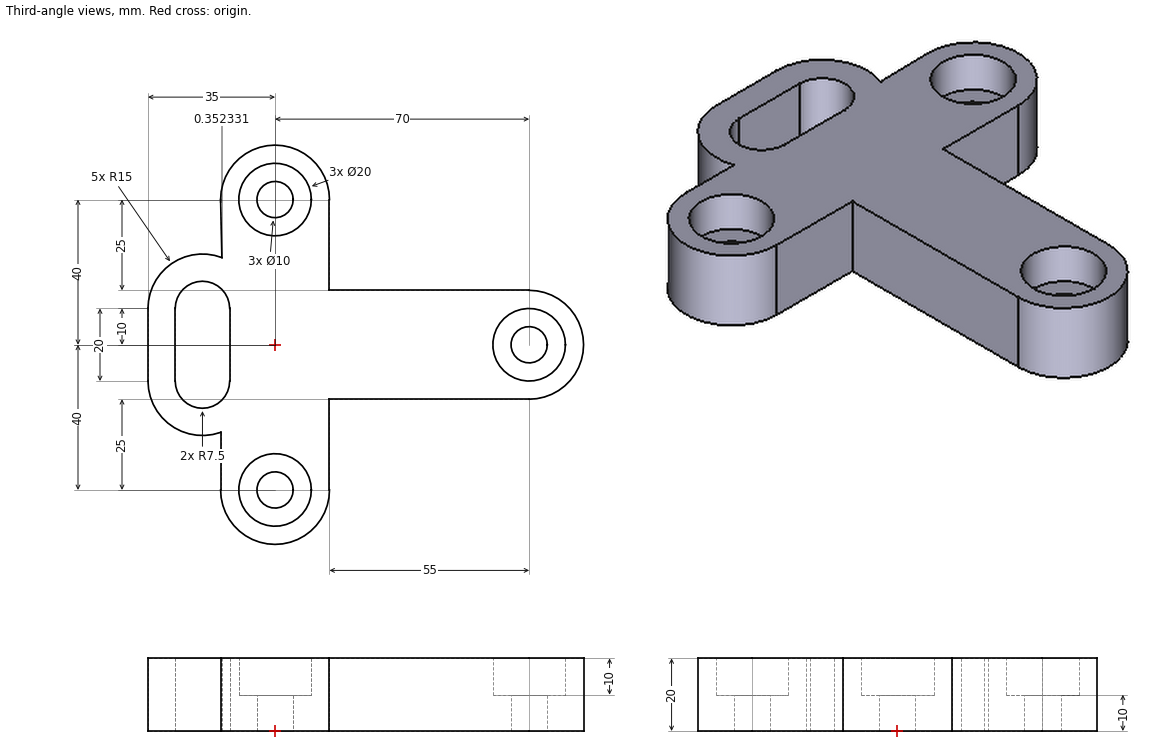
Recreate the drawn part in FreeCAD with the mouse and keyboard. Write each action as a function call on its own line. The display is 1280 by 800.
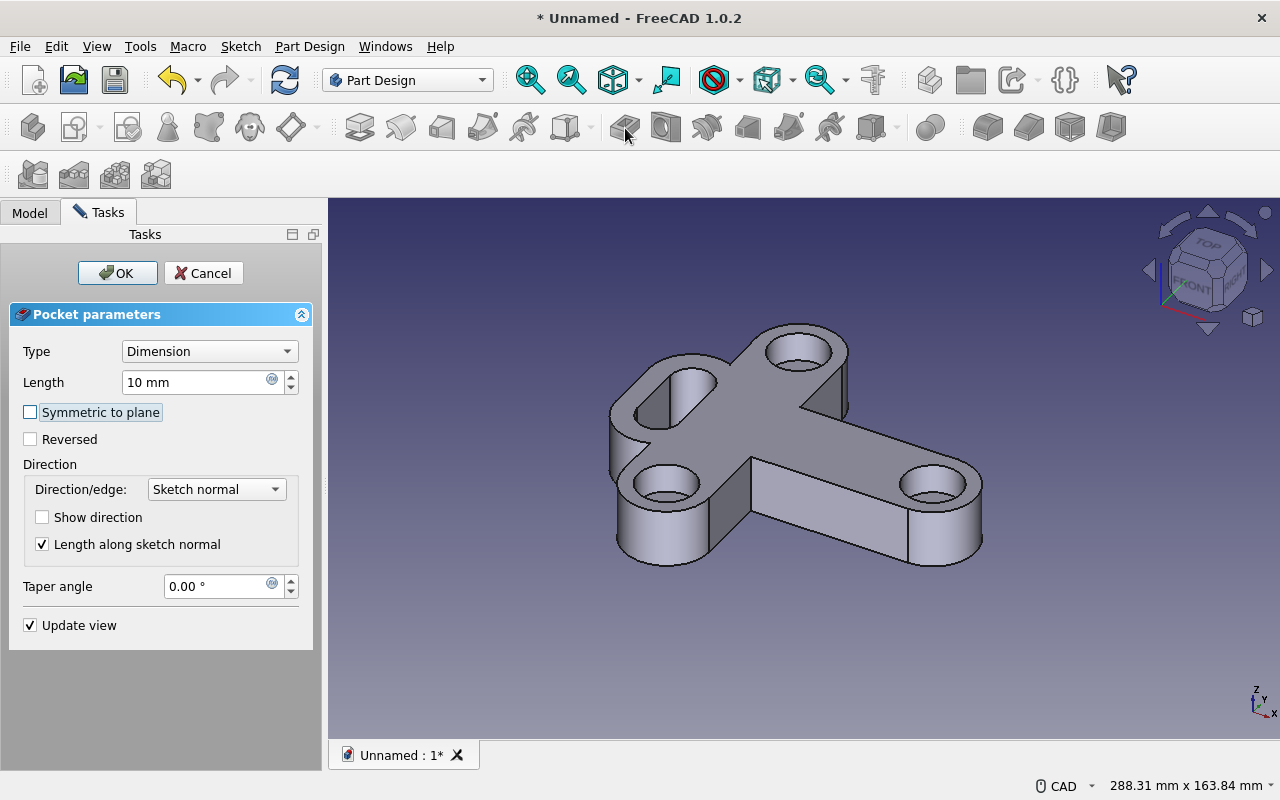
click(118, 273)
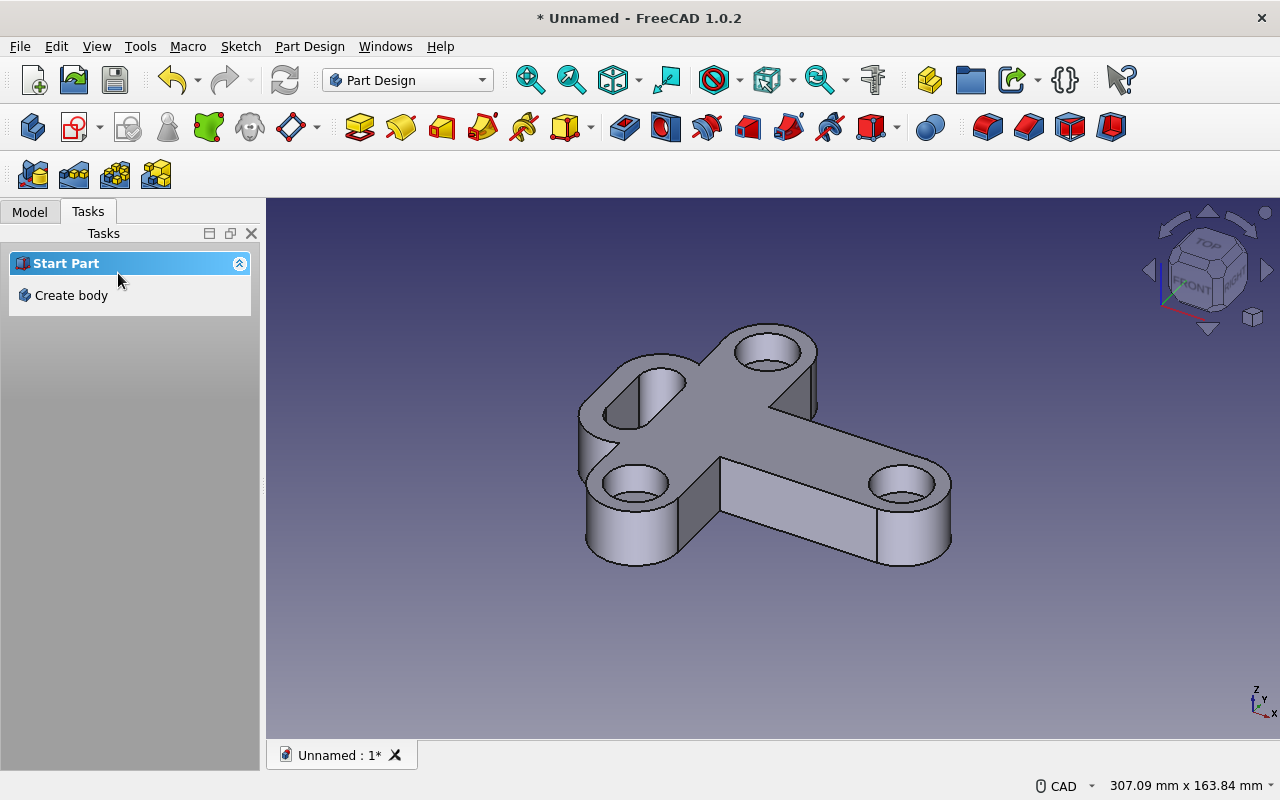
key(0)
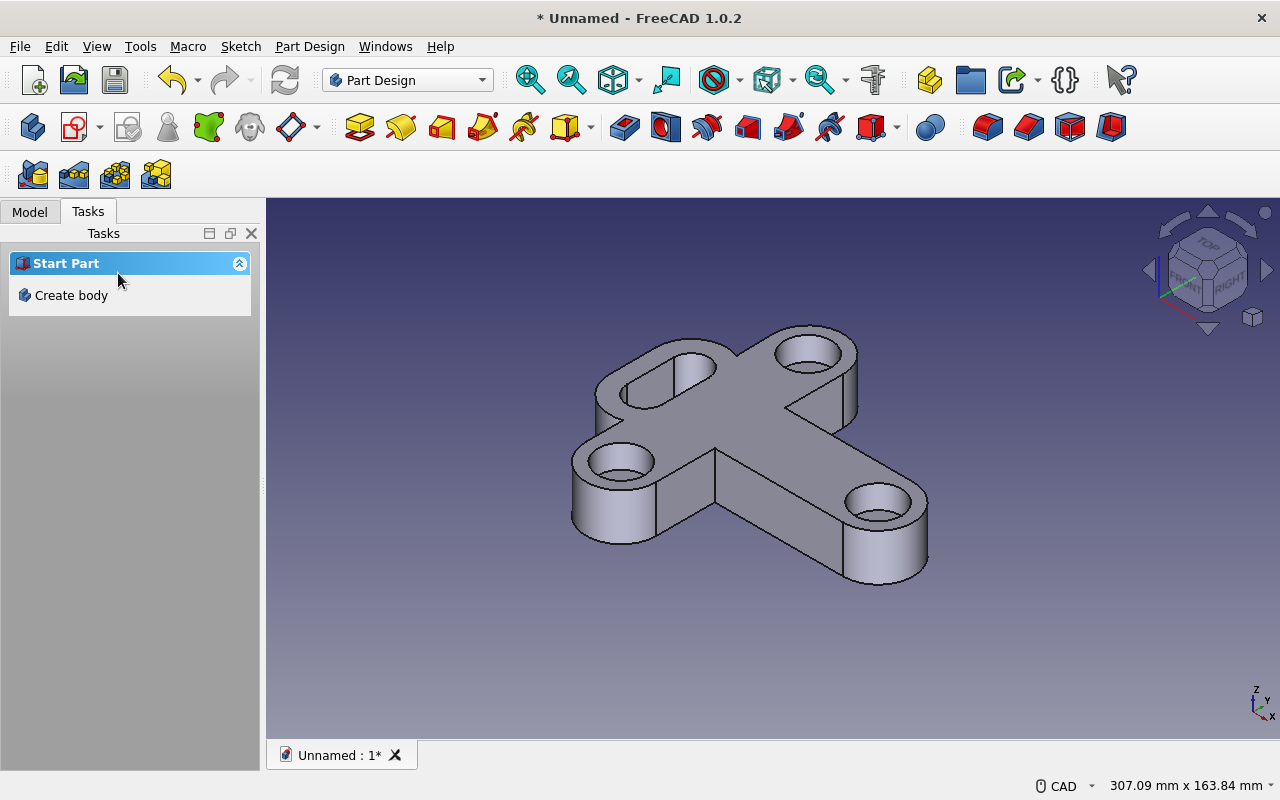
key(2)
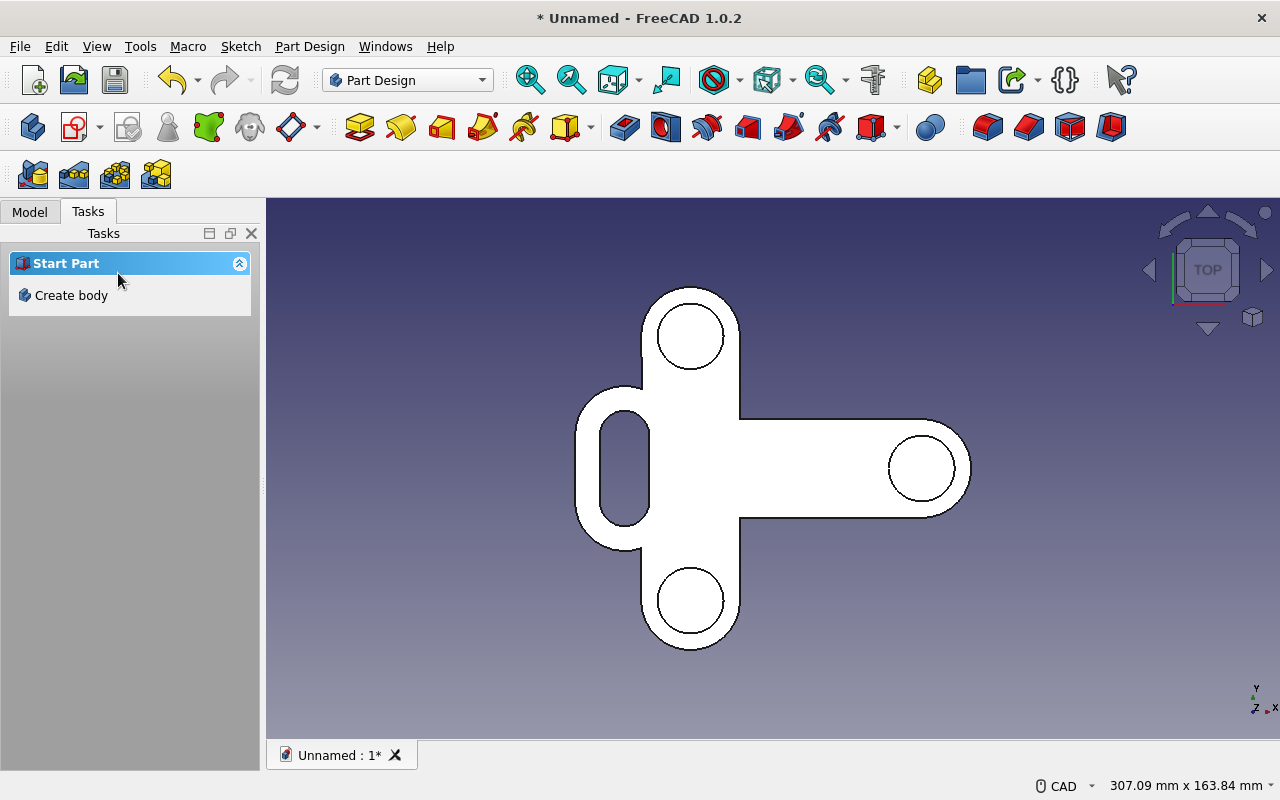
click(922, 467)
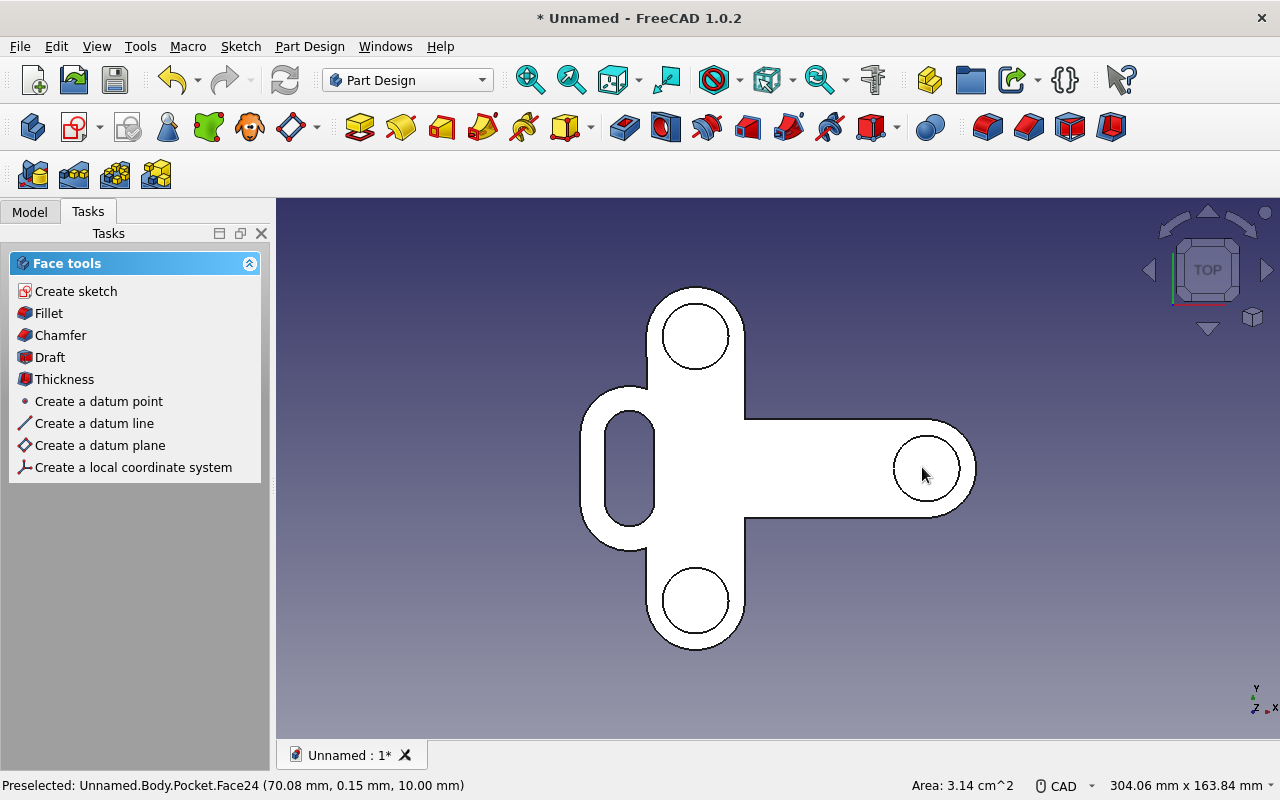
click(74, 128)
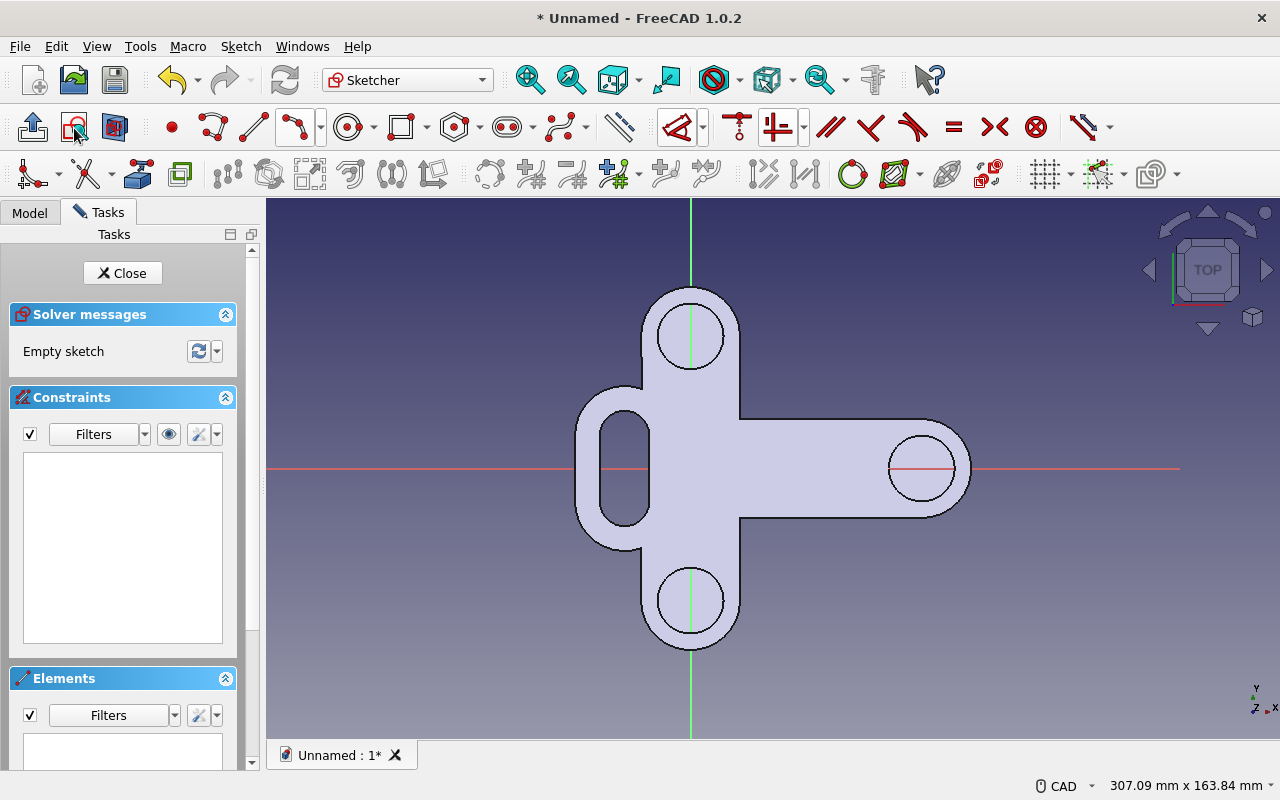
click(348, 128)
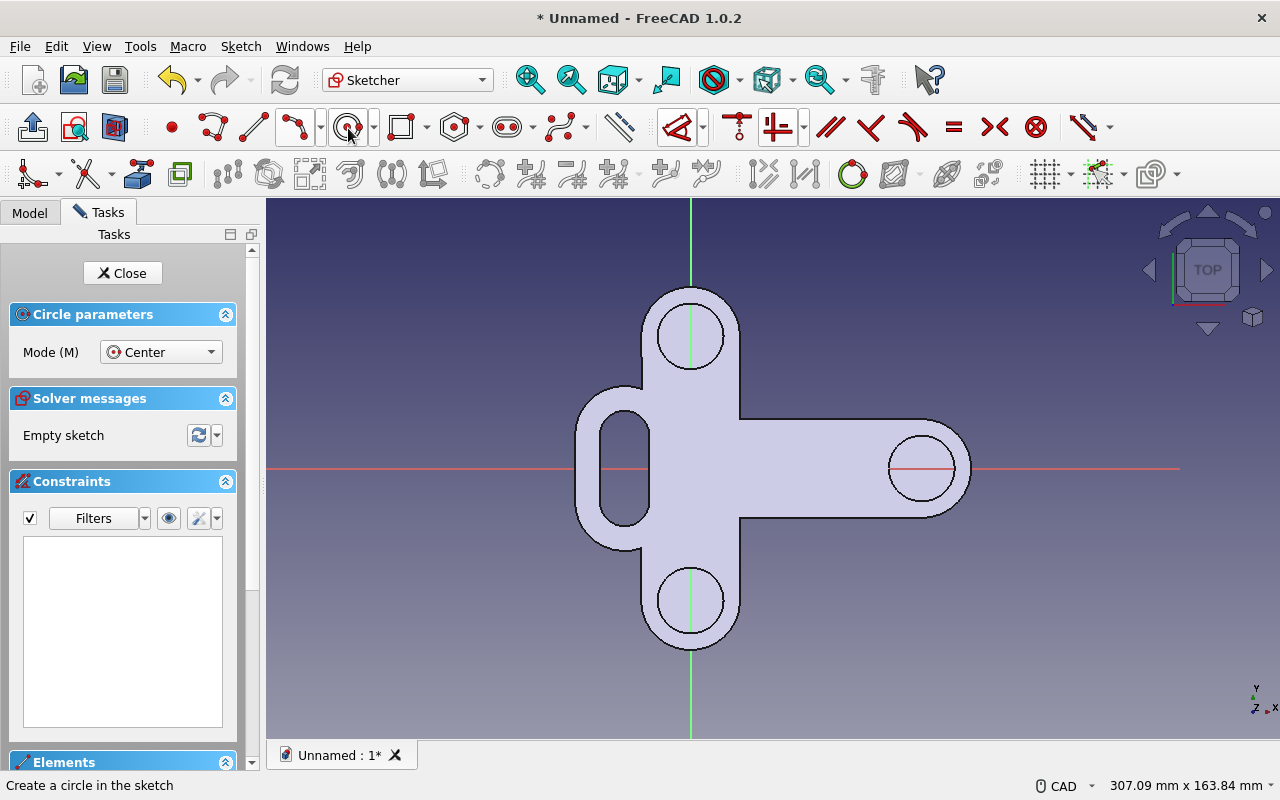
scroll(691, 336, up, 2)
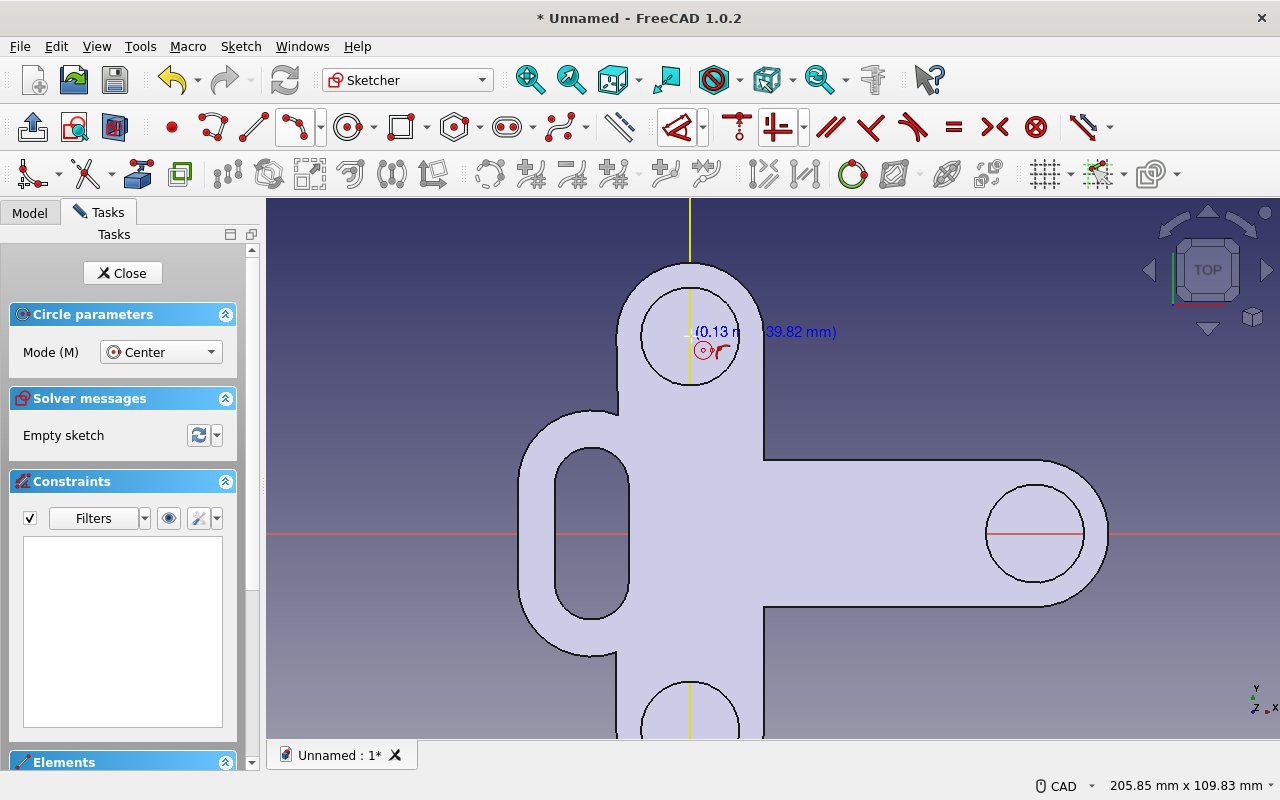
click(690, 337)
move(708, 319)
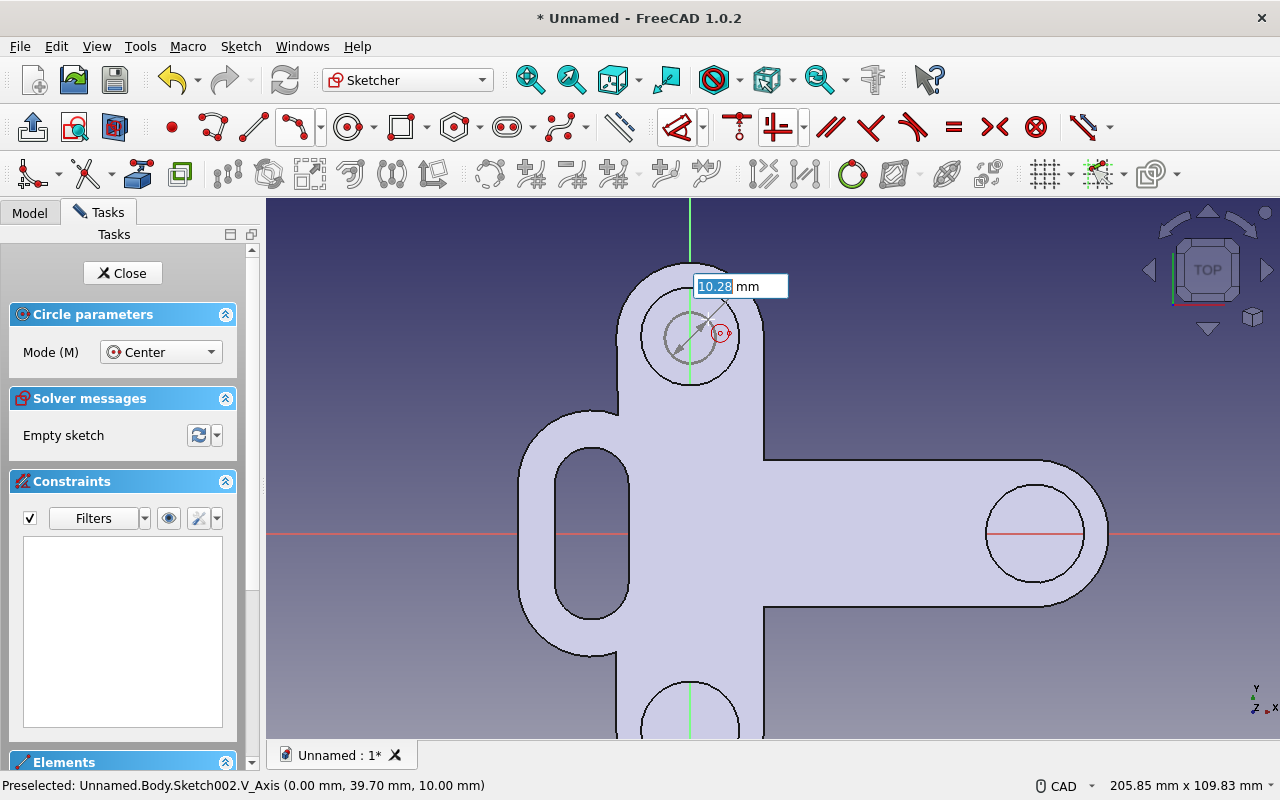
text(10)
key(Return)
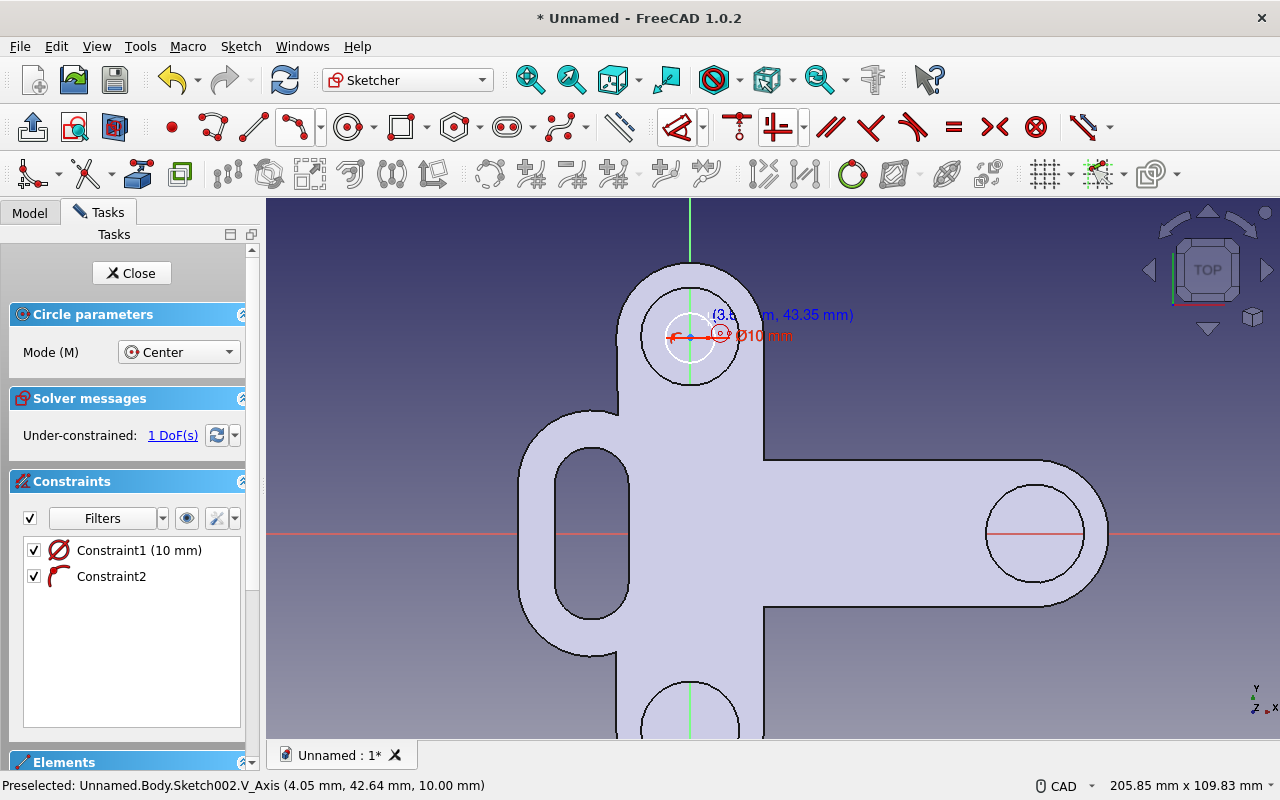
scroll(294, 226, down, 1)